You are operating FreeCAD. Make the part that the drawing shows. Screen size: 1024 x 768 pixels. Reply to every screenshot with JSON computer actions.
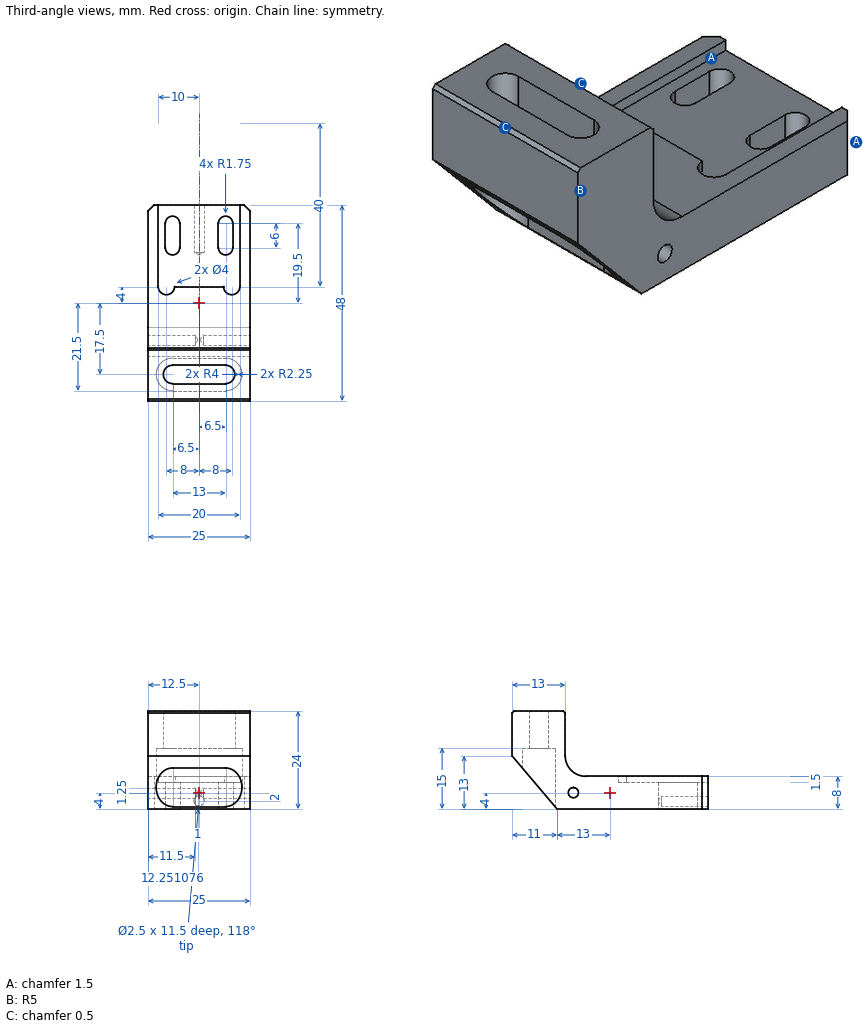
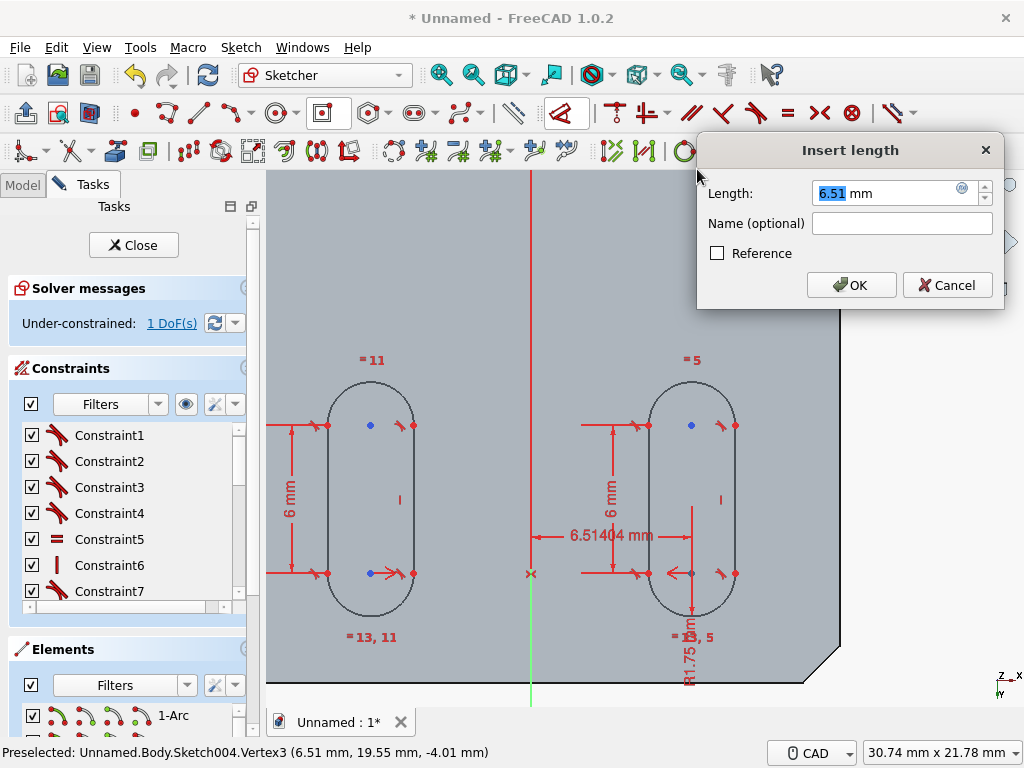
{"action": "type", "text": "6.5"}
{"action": "key", "text": "Return"}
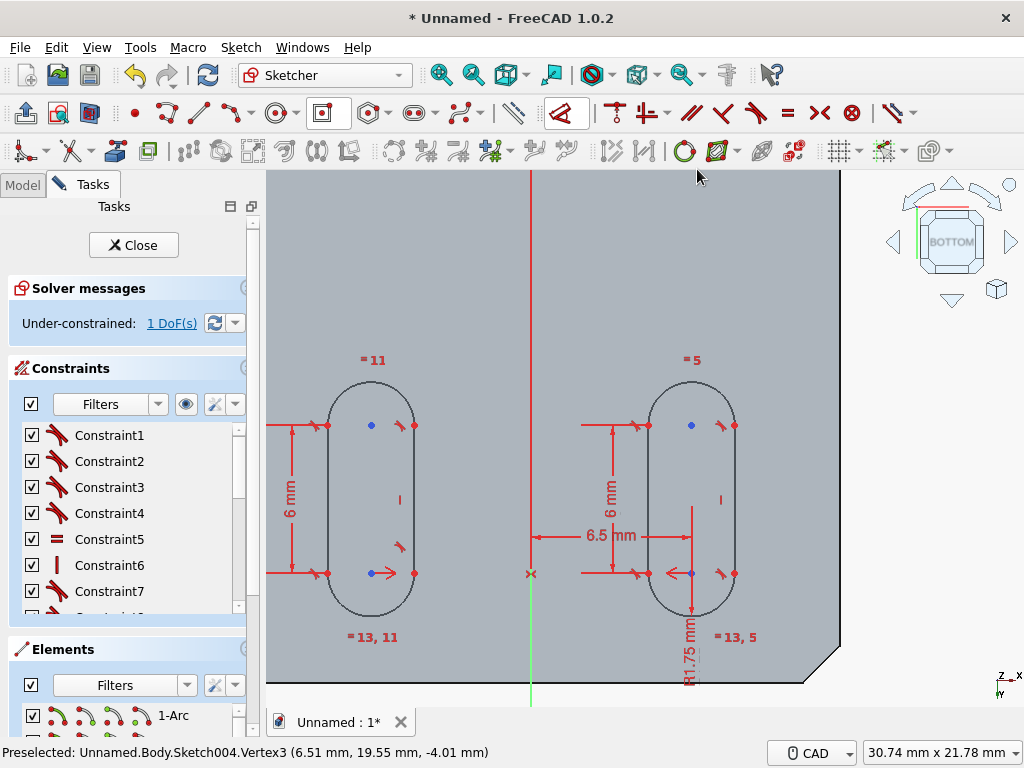
{"action": "left_click", "coordinate": [648, 573]}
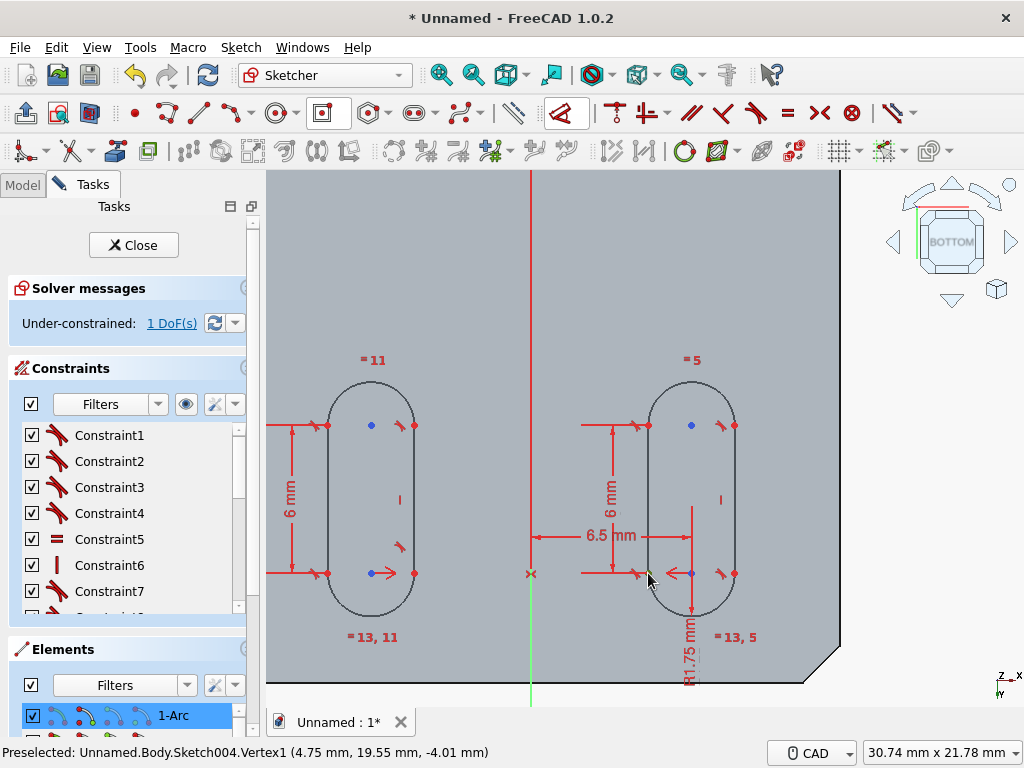
{"action": "left_click", "coordinate": [584, 114]}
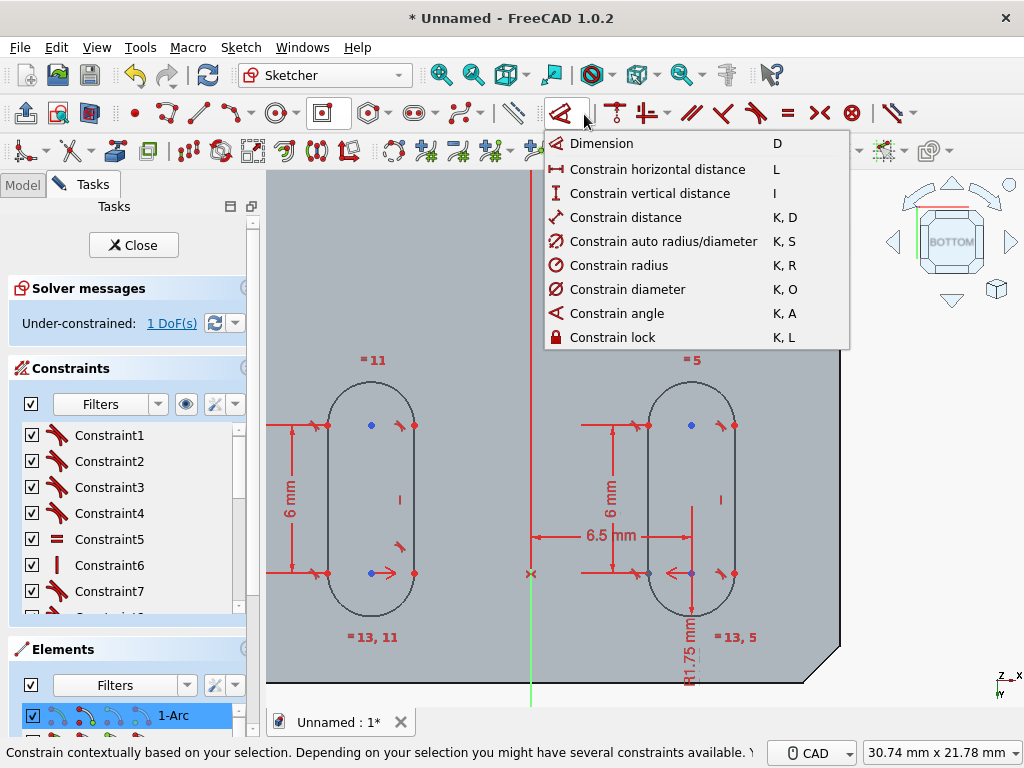
{"action": "left_click", "coordinate": [697, 193]}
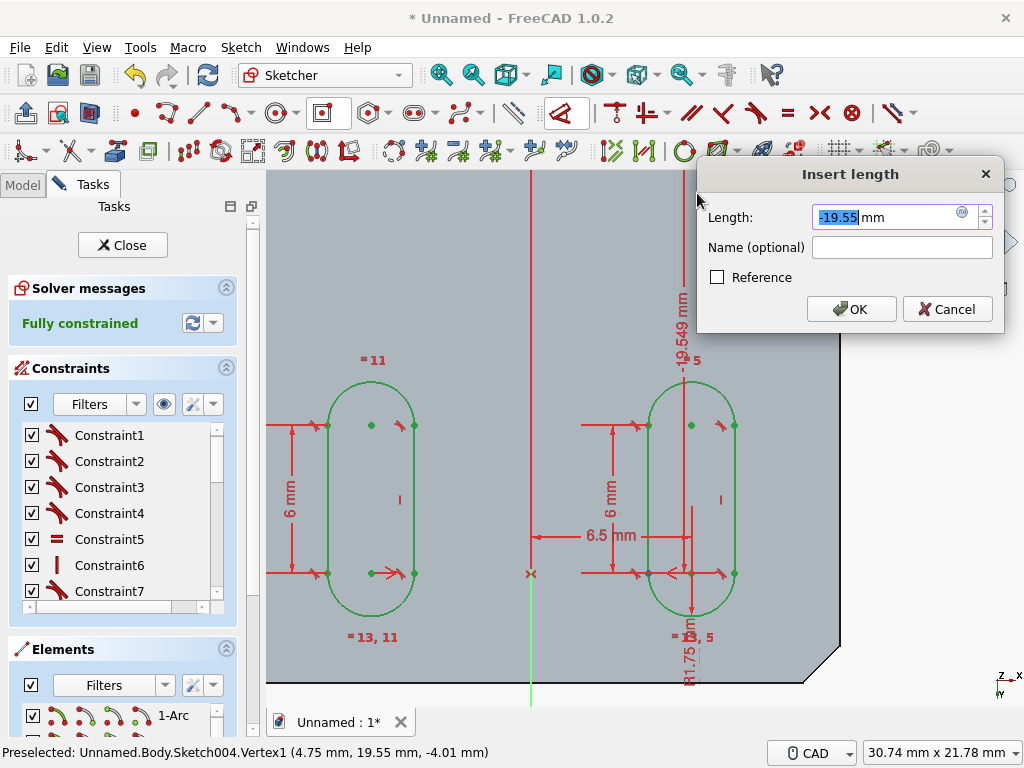
{"action": "type", "text": "-19.5"}
{"action": "key", "text": "Return"}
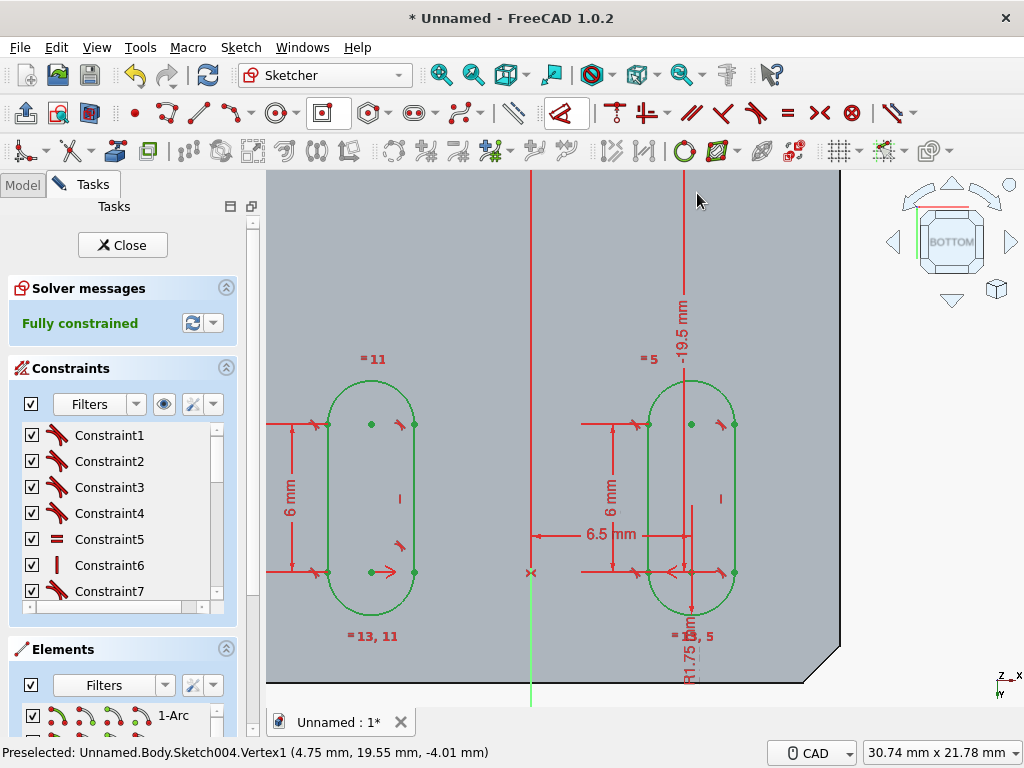
{"action": "left_click", "coordinate": [123, 245]}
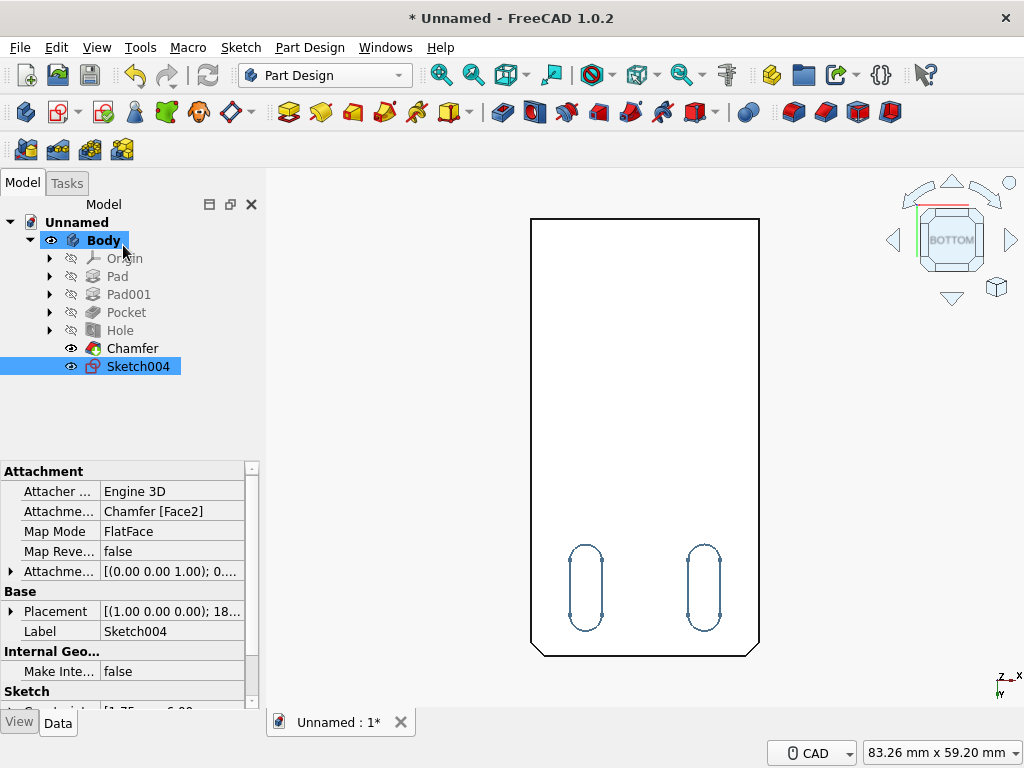
{"action": "left_click", "coordinate": [504, 112]}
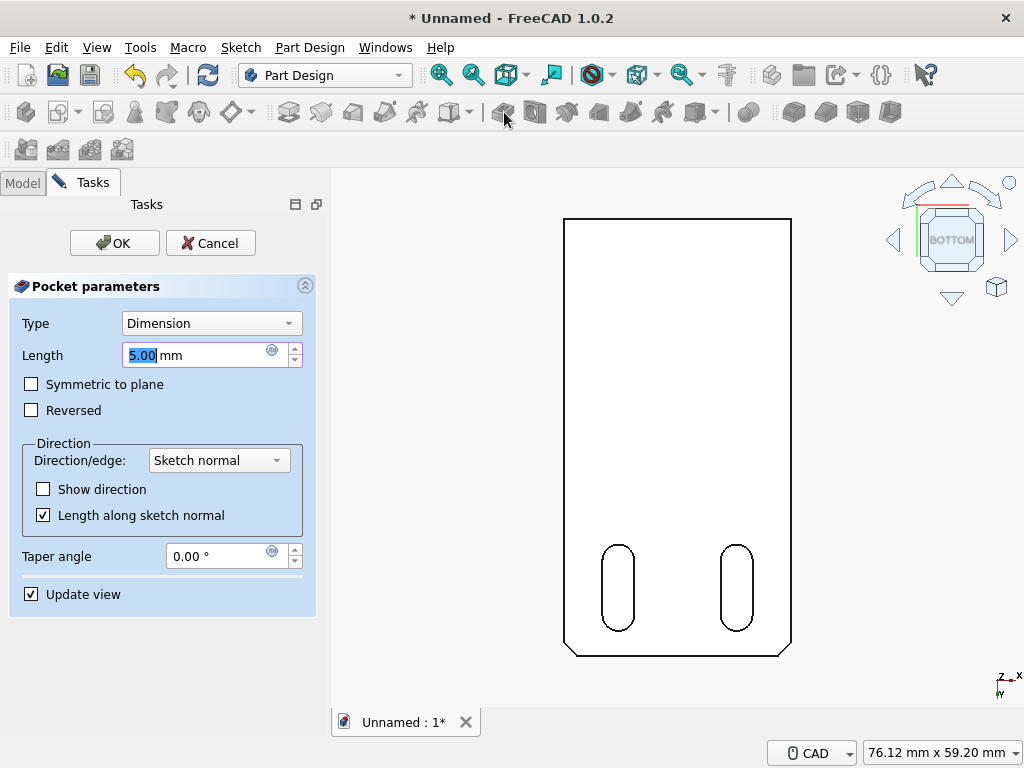
{"action": "left_click", "coordinate": [212, 324]}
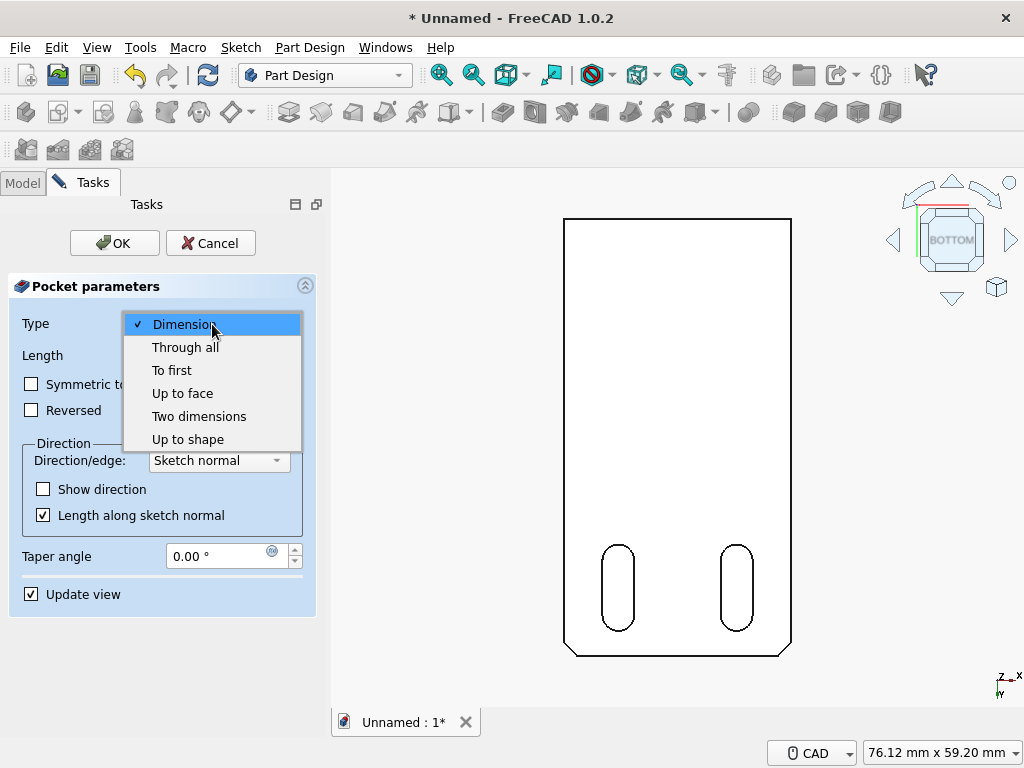
{"action": "left_click", "coordinate": [212, 348]}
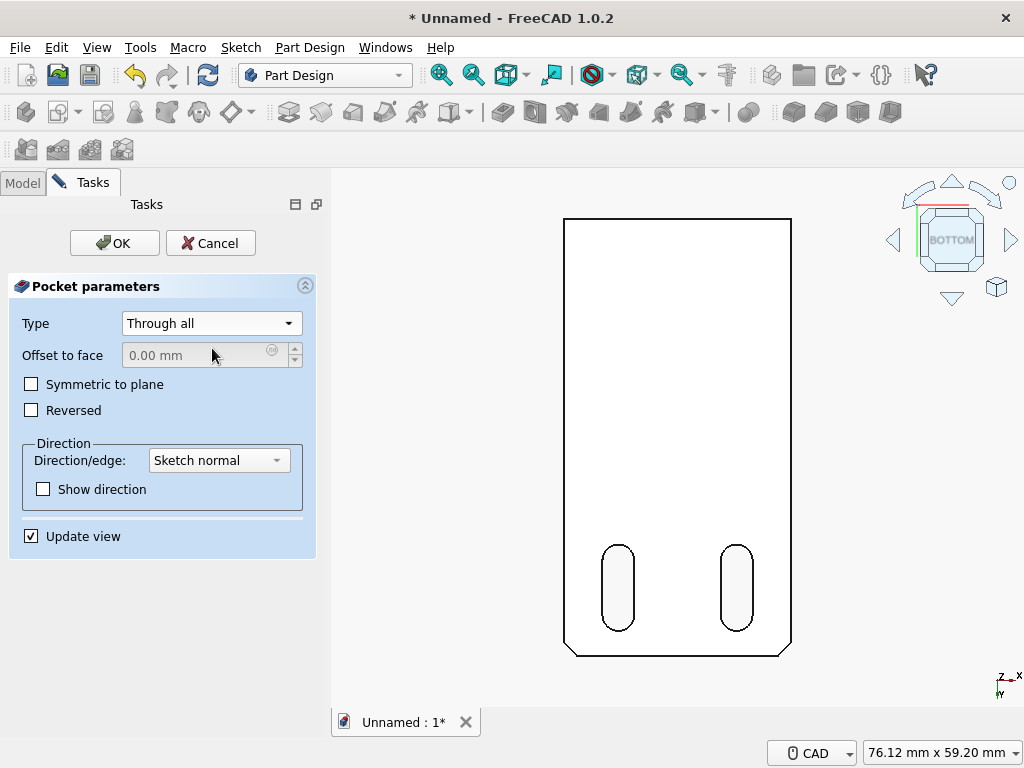
{"action": "left_click", "coordinate": [115, 243]}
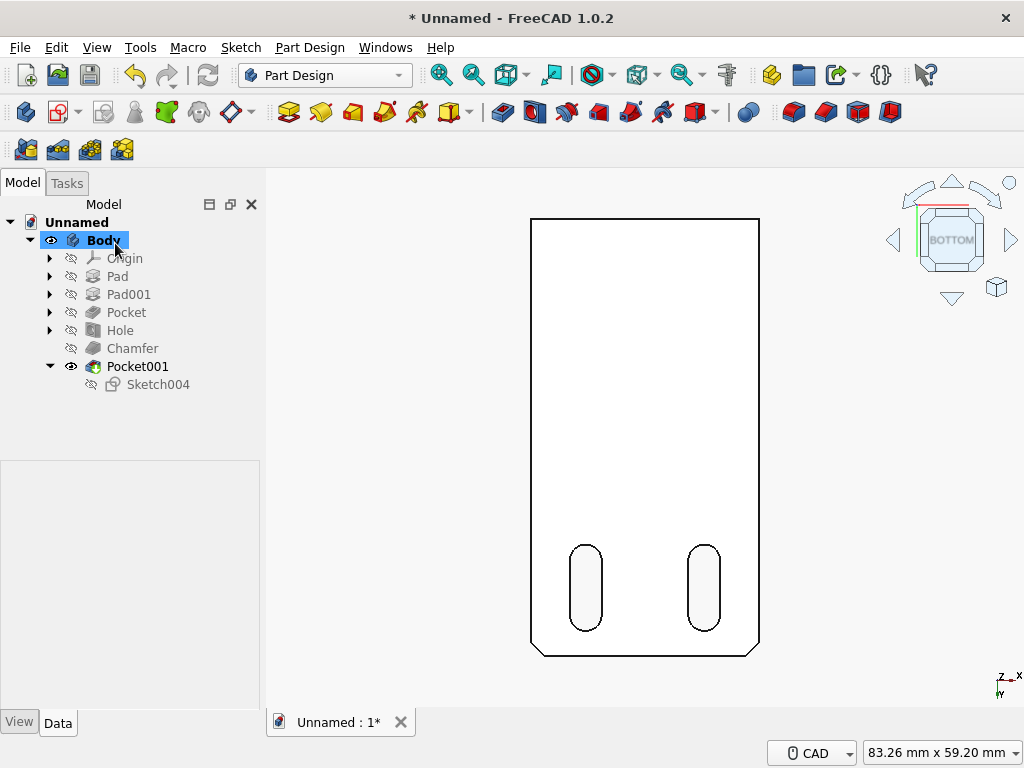
{"action": "left_click", "coordinate": [50, 258]}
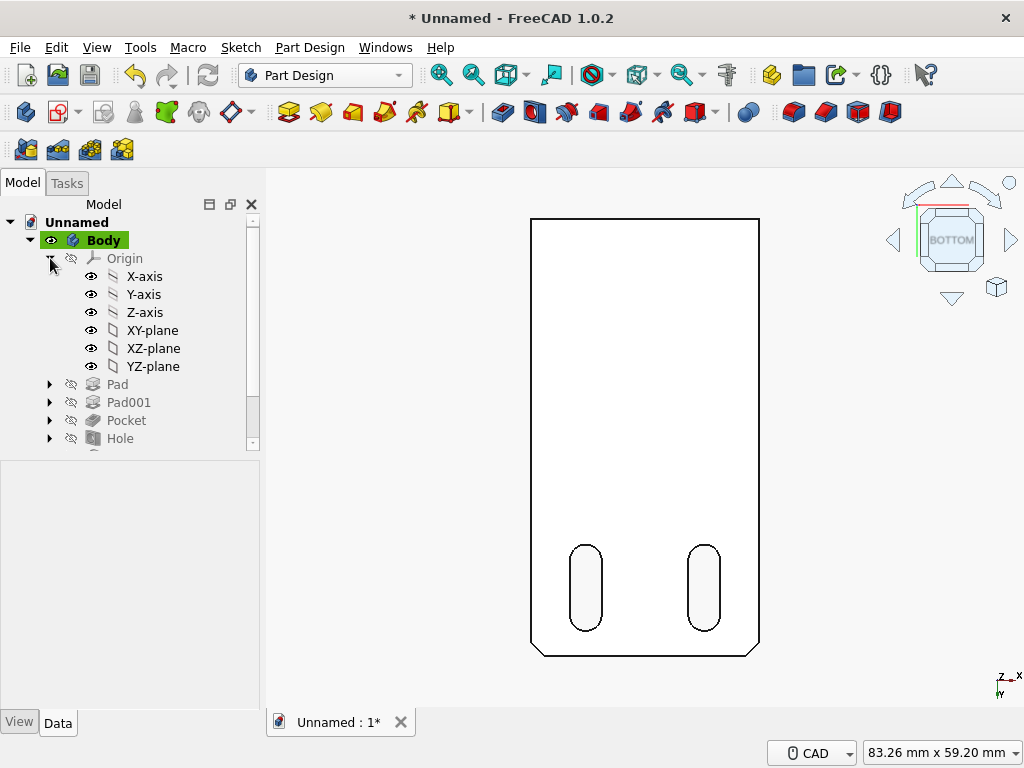
{"action": "left_click", "coordinate": [136, 348]}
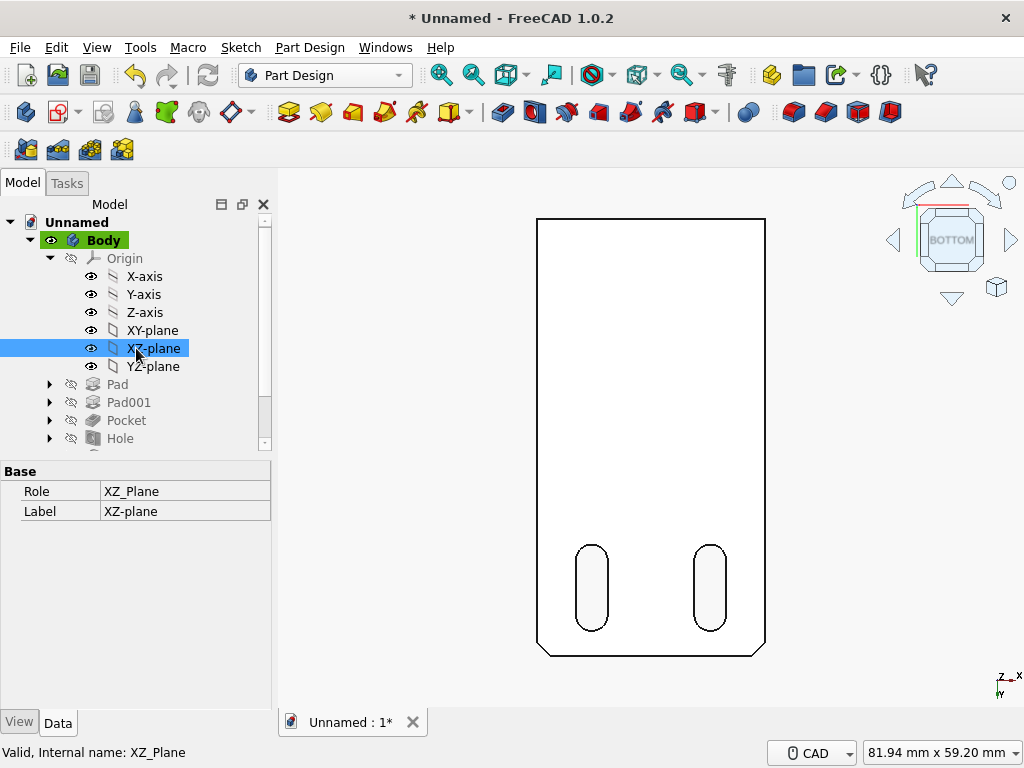
{"action": "left_click", "coordinate": [232, 112]}